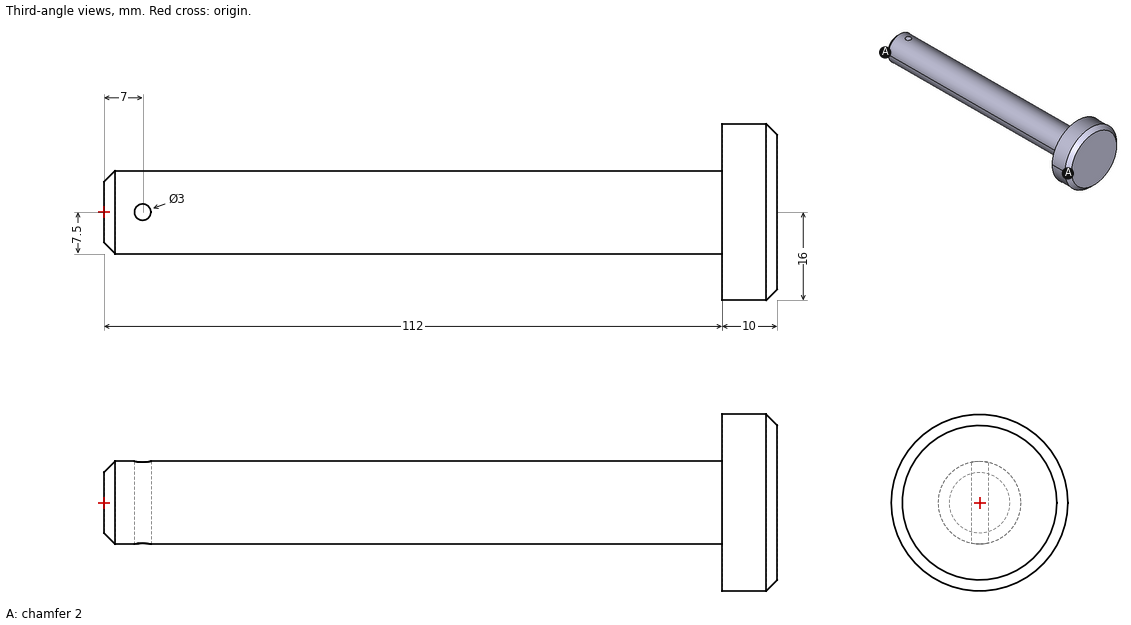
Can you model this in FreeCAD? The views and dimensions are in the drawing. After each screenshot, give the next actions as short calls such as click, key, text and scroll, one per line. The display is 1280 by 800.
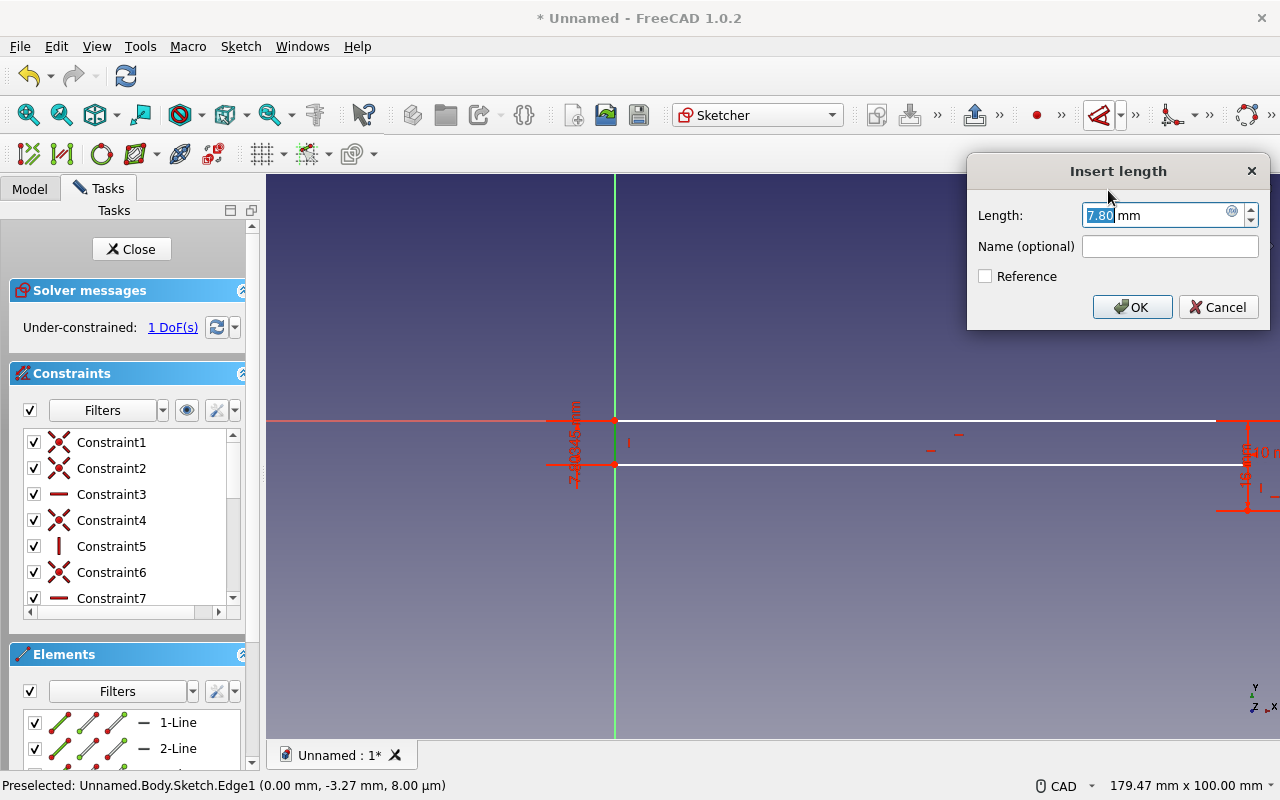
text(7.5)
key(Return)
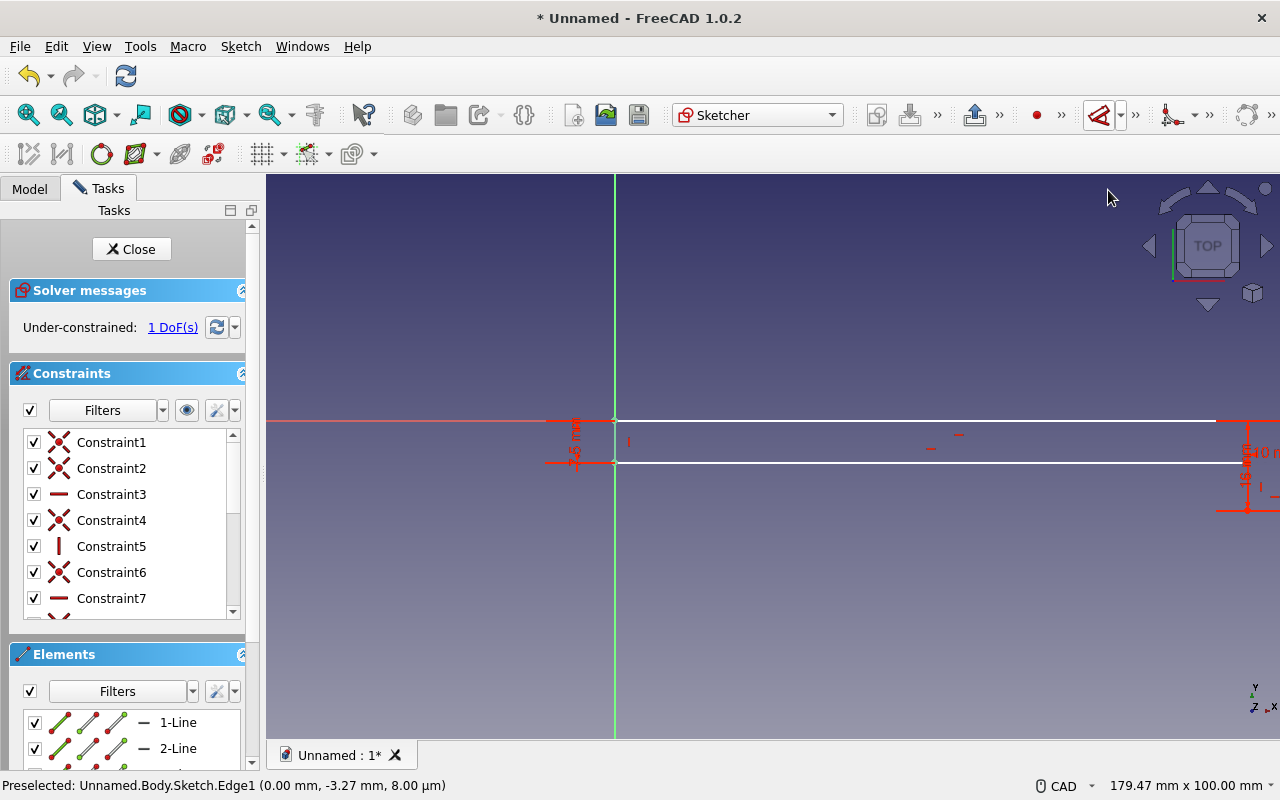
click(805, 463)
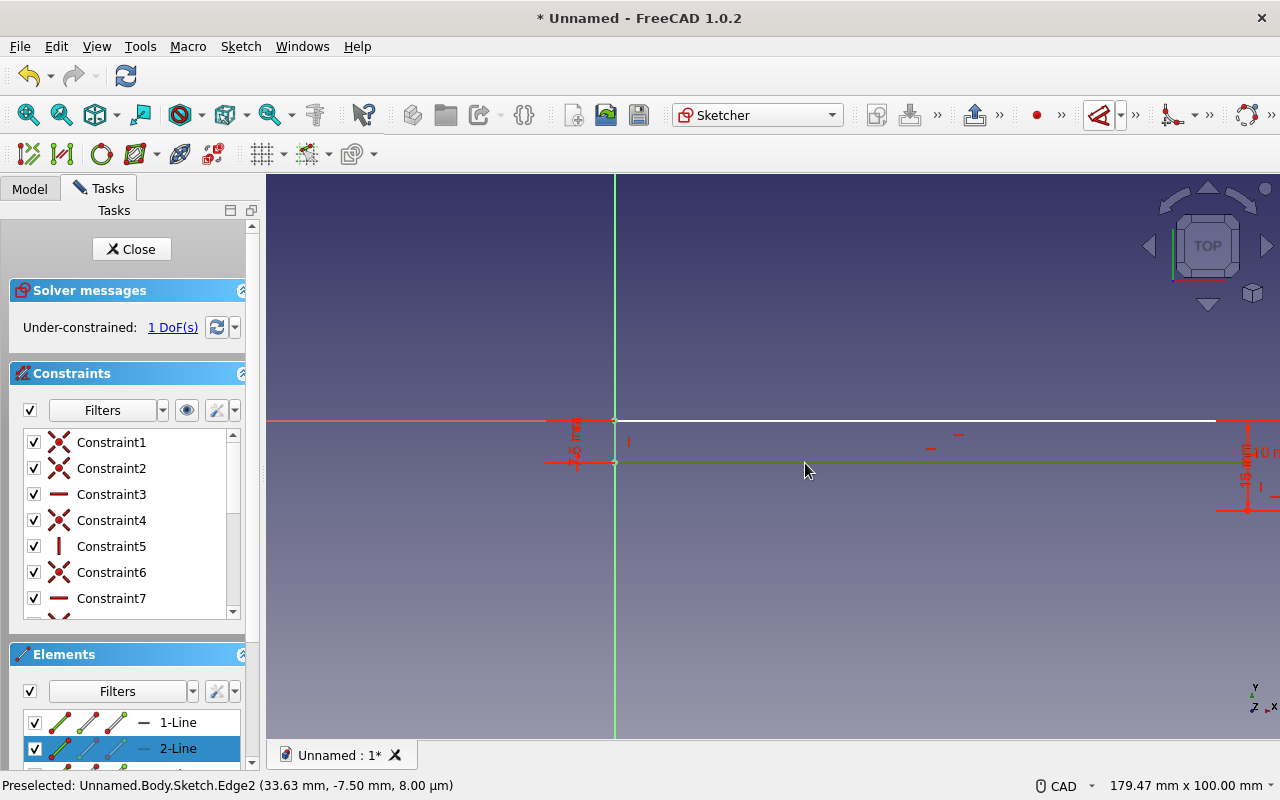
click(1120, 116)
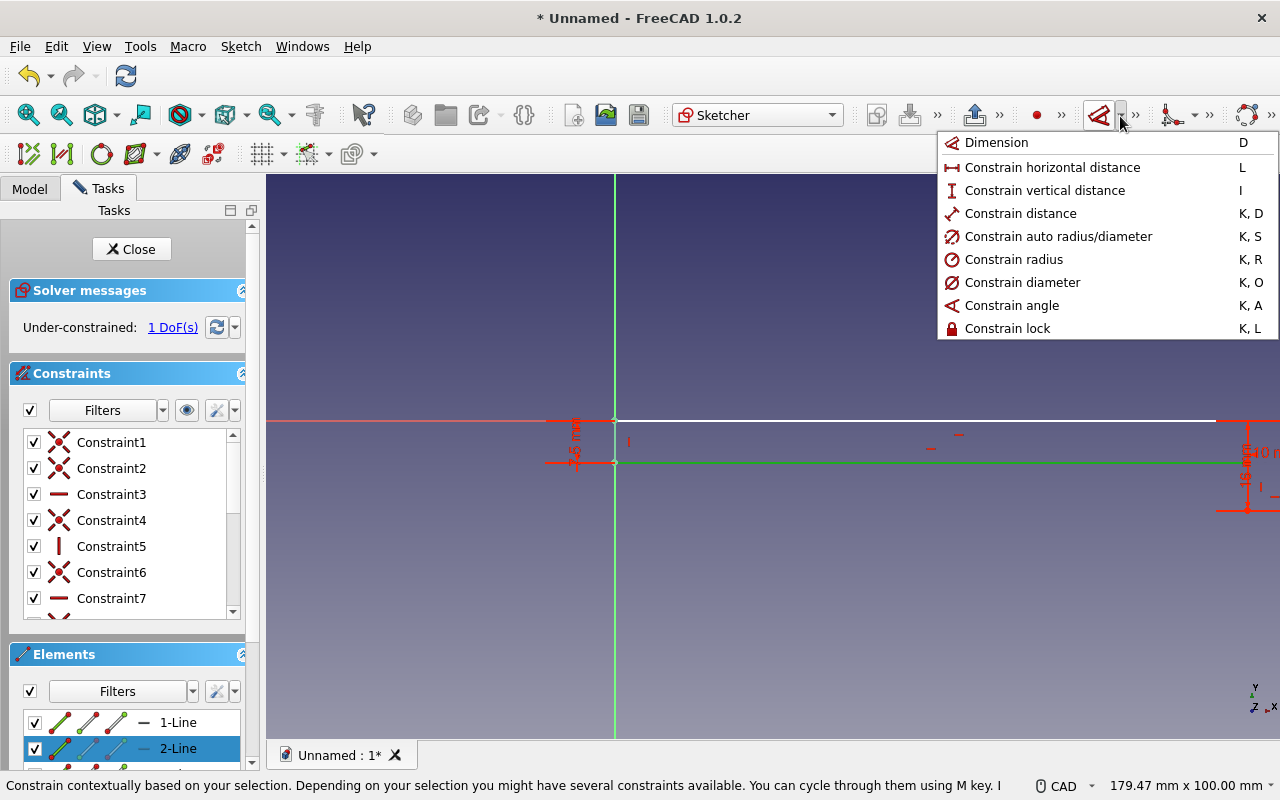
click(1108, 168)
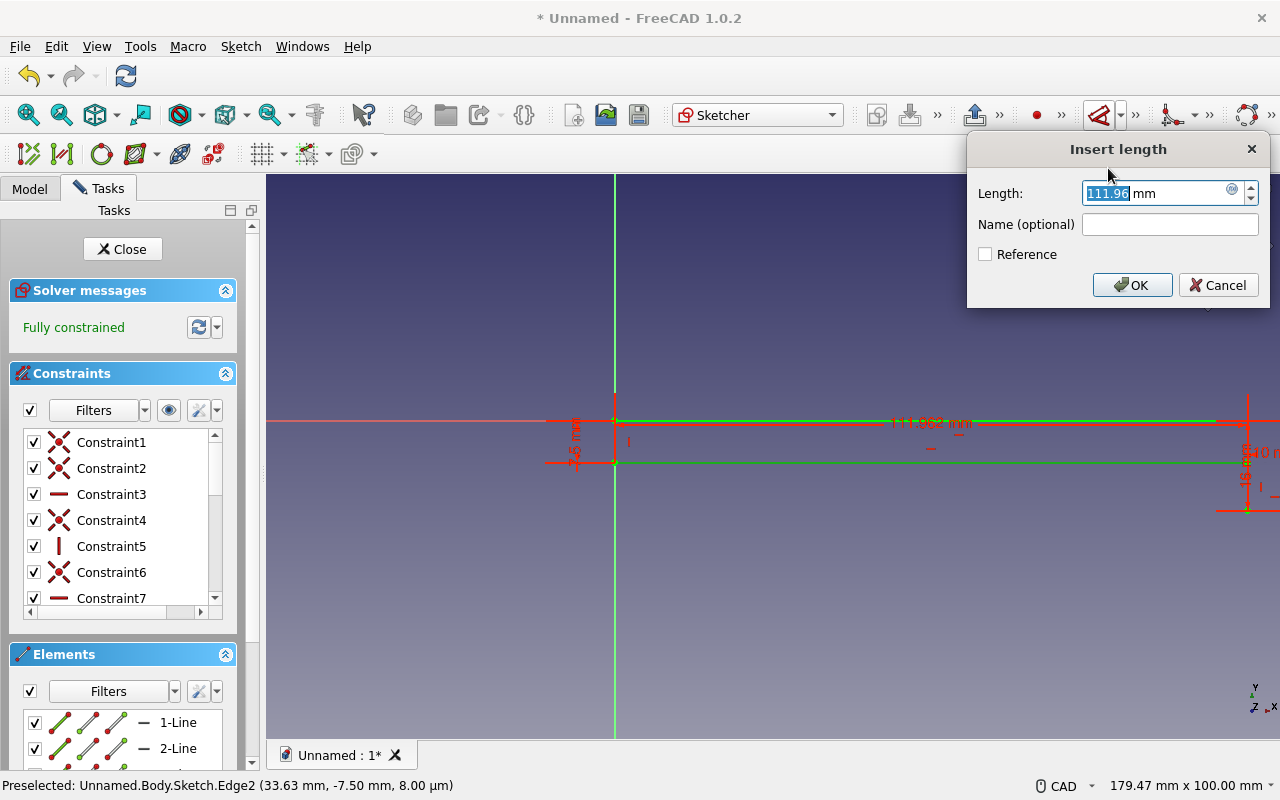
text(112)
key(Return)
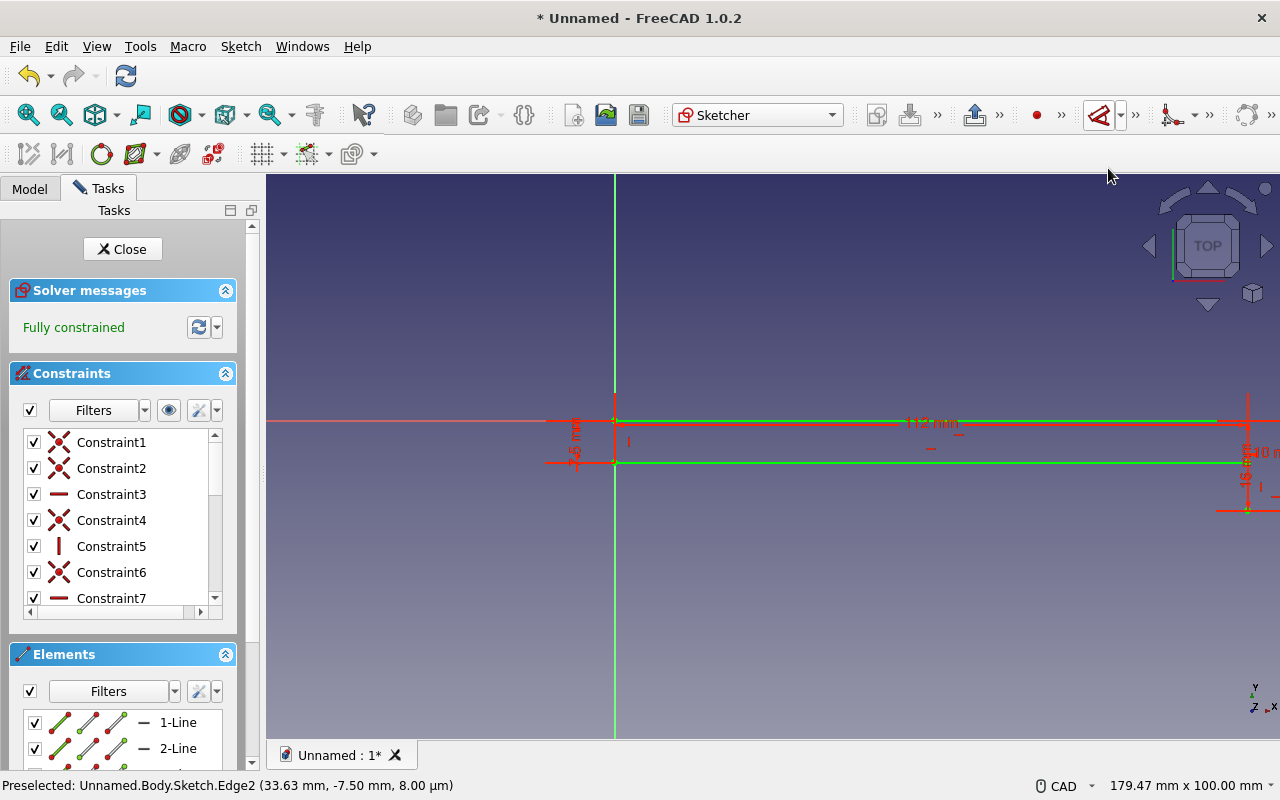
click(123, 249)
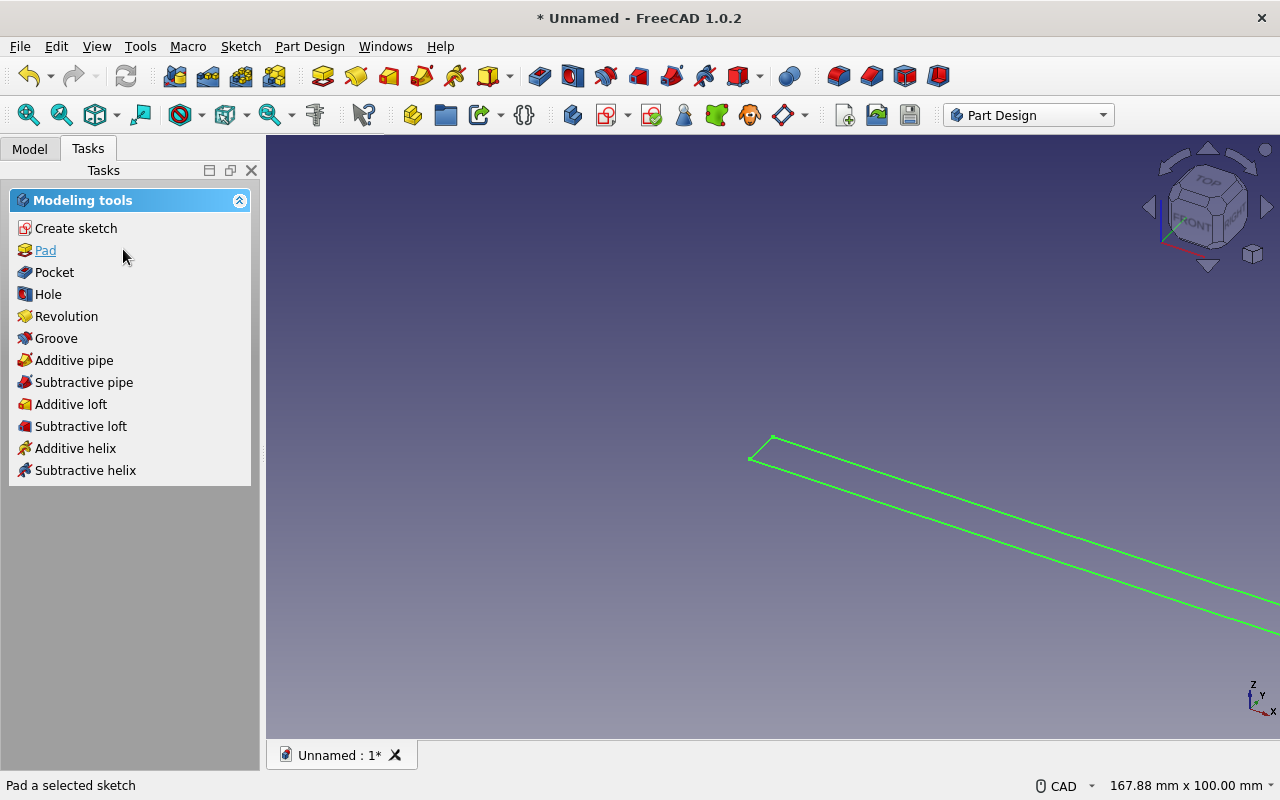
click(356, 76)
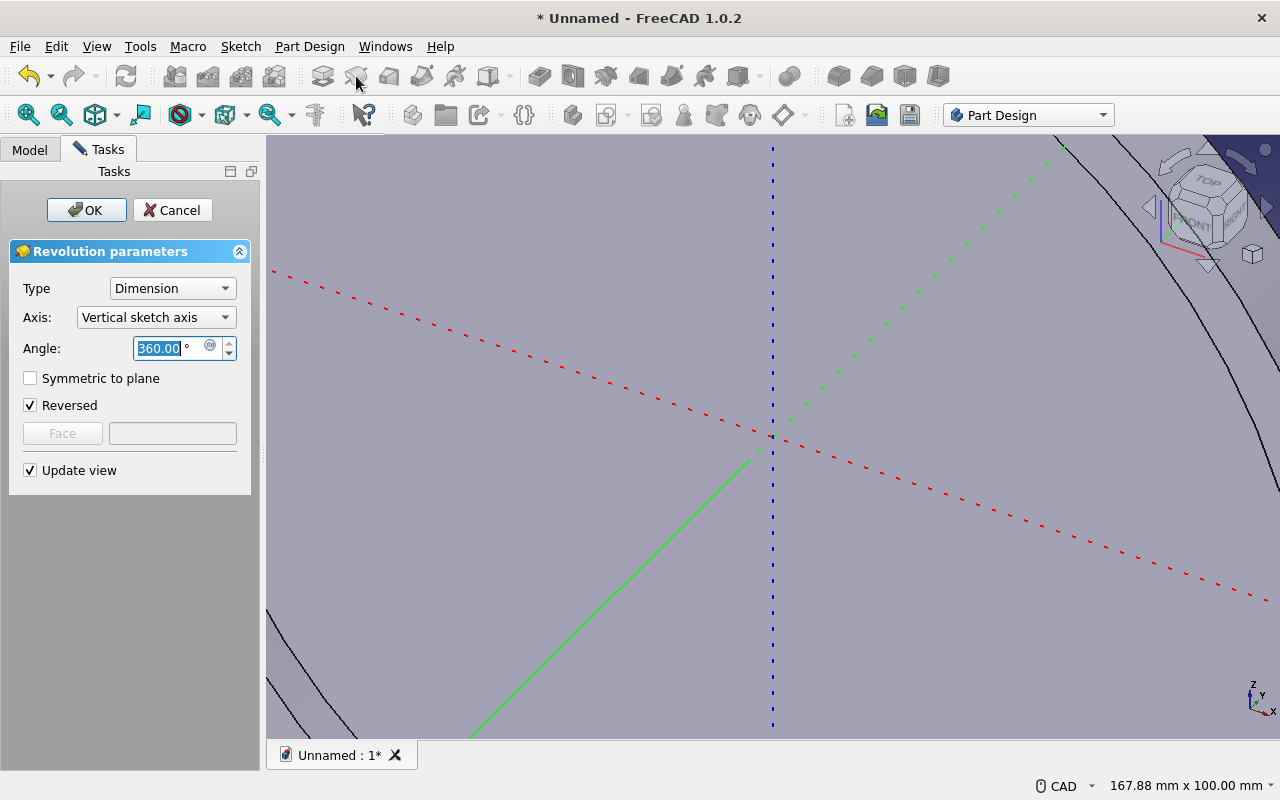
click(157, 318)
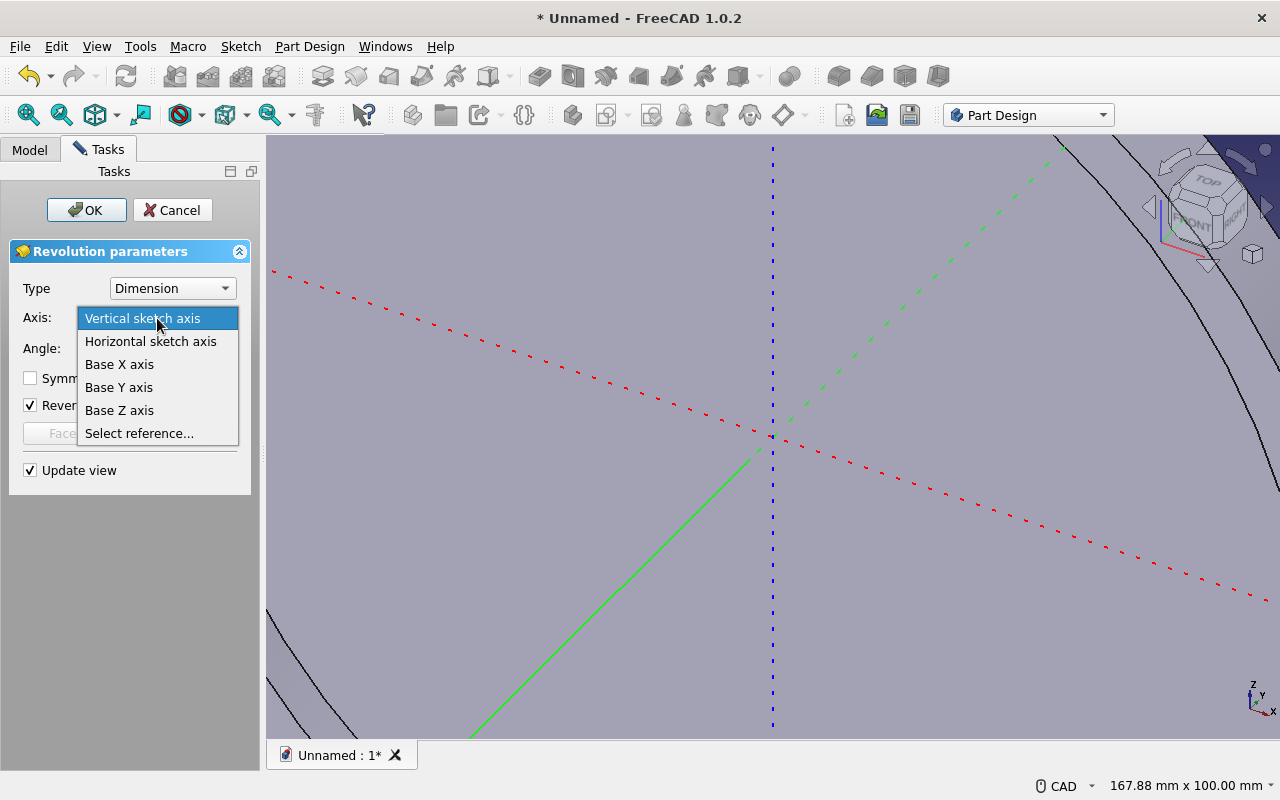
click(156, 342)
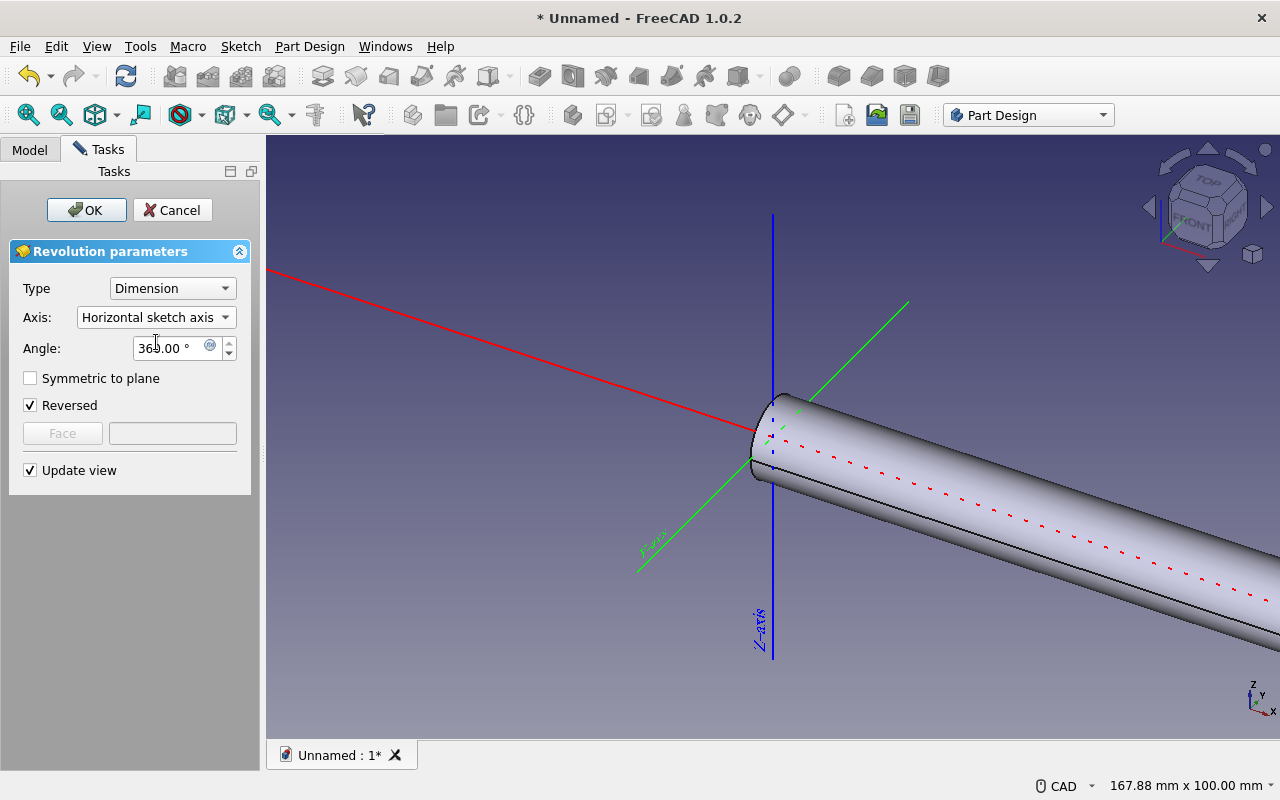
click(87, 210)